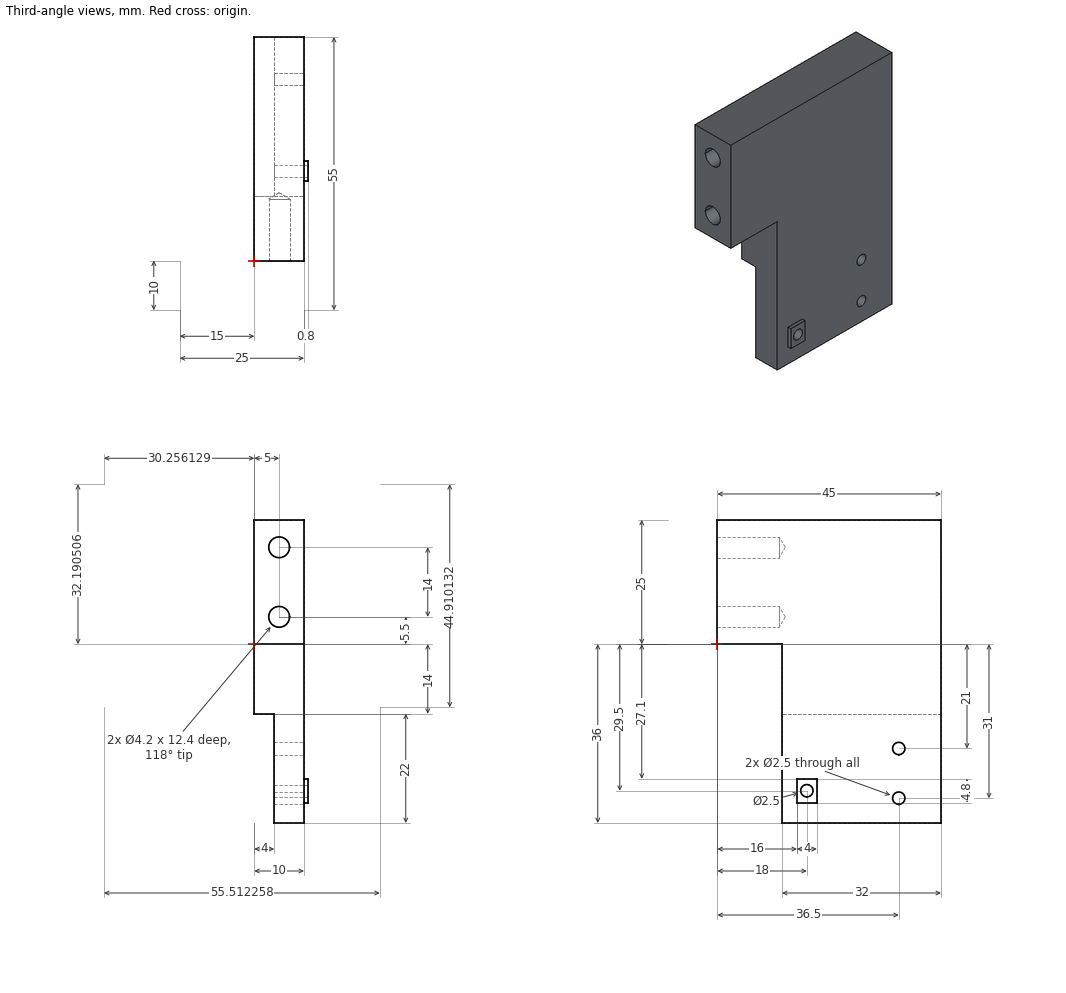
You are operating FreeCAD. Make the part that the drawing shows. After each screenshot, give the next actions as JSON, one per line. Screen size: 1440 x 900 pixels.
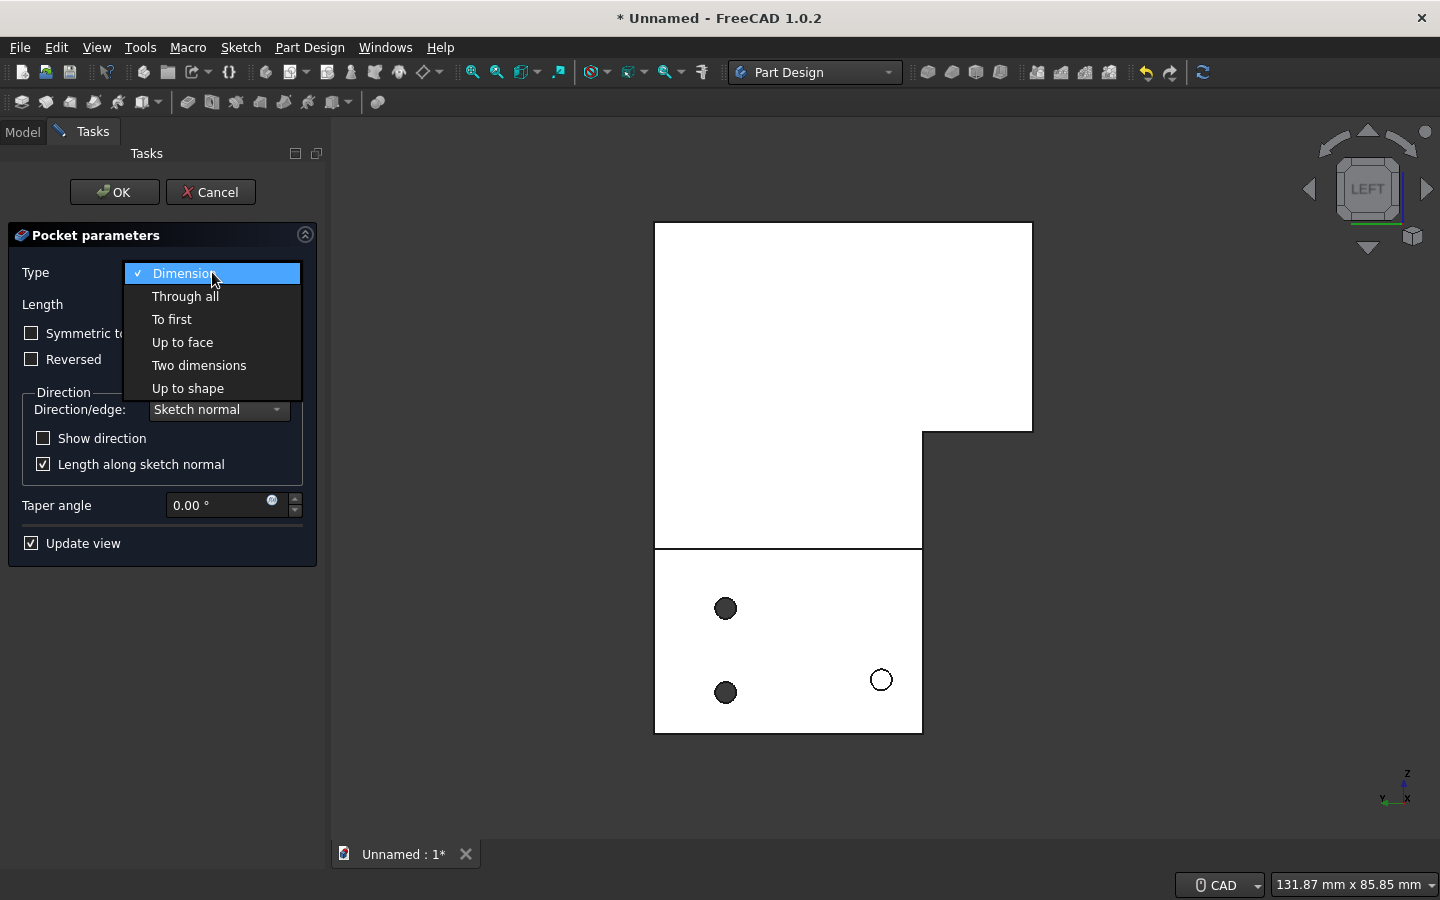
{"action": "left_click", "coordinate": [212, 296]}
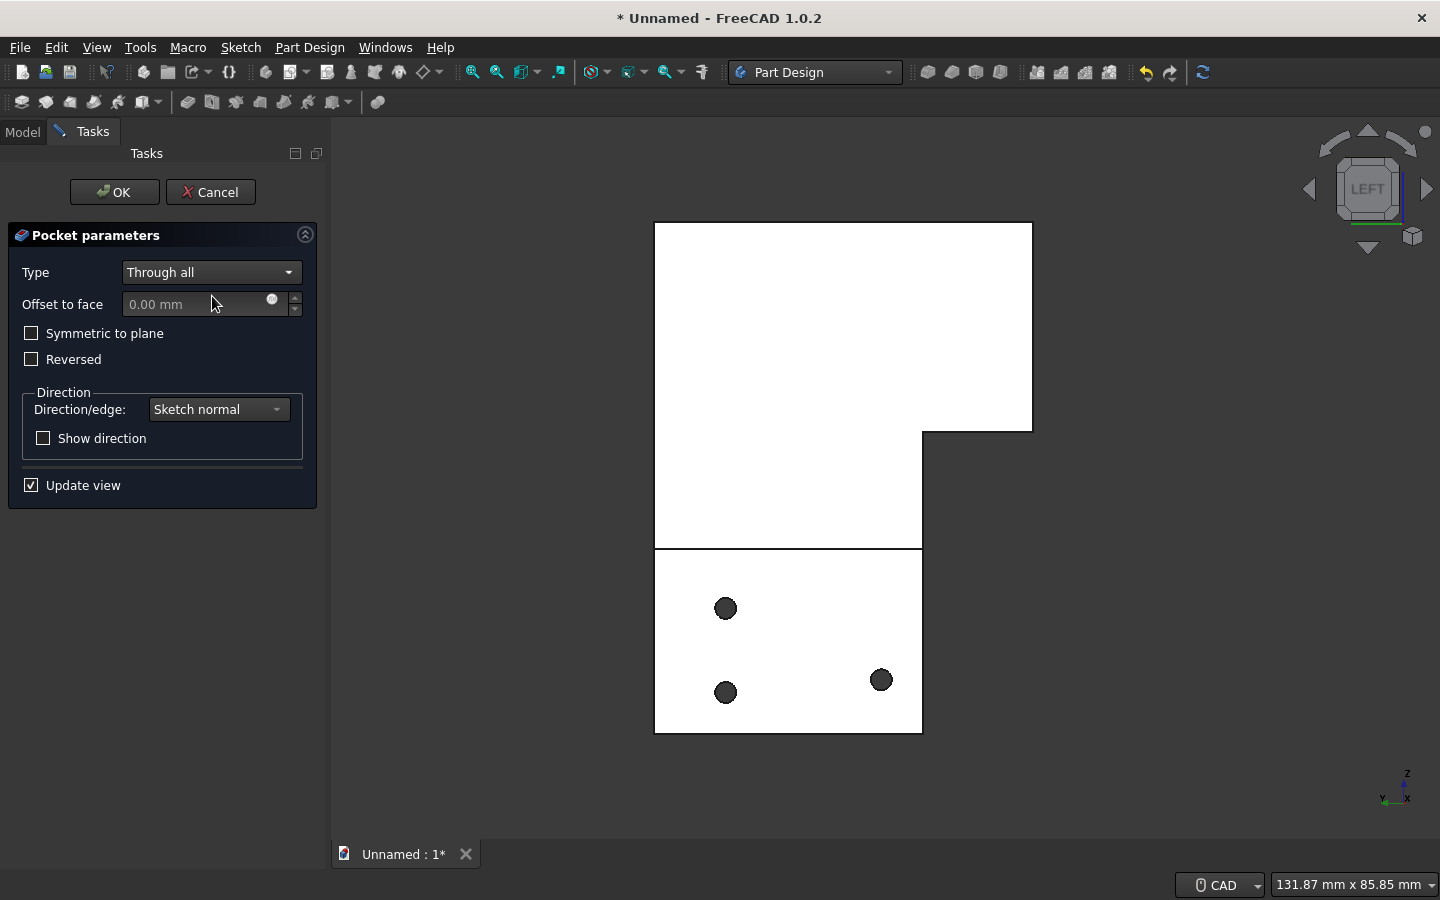
{"action": "left_click", "coordinate": [115, 192]}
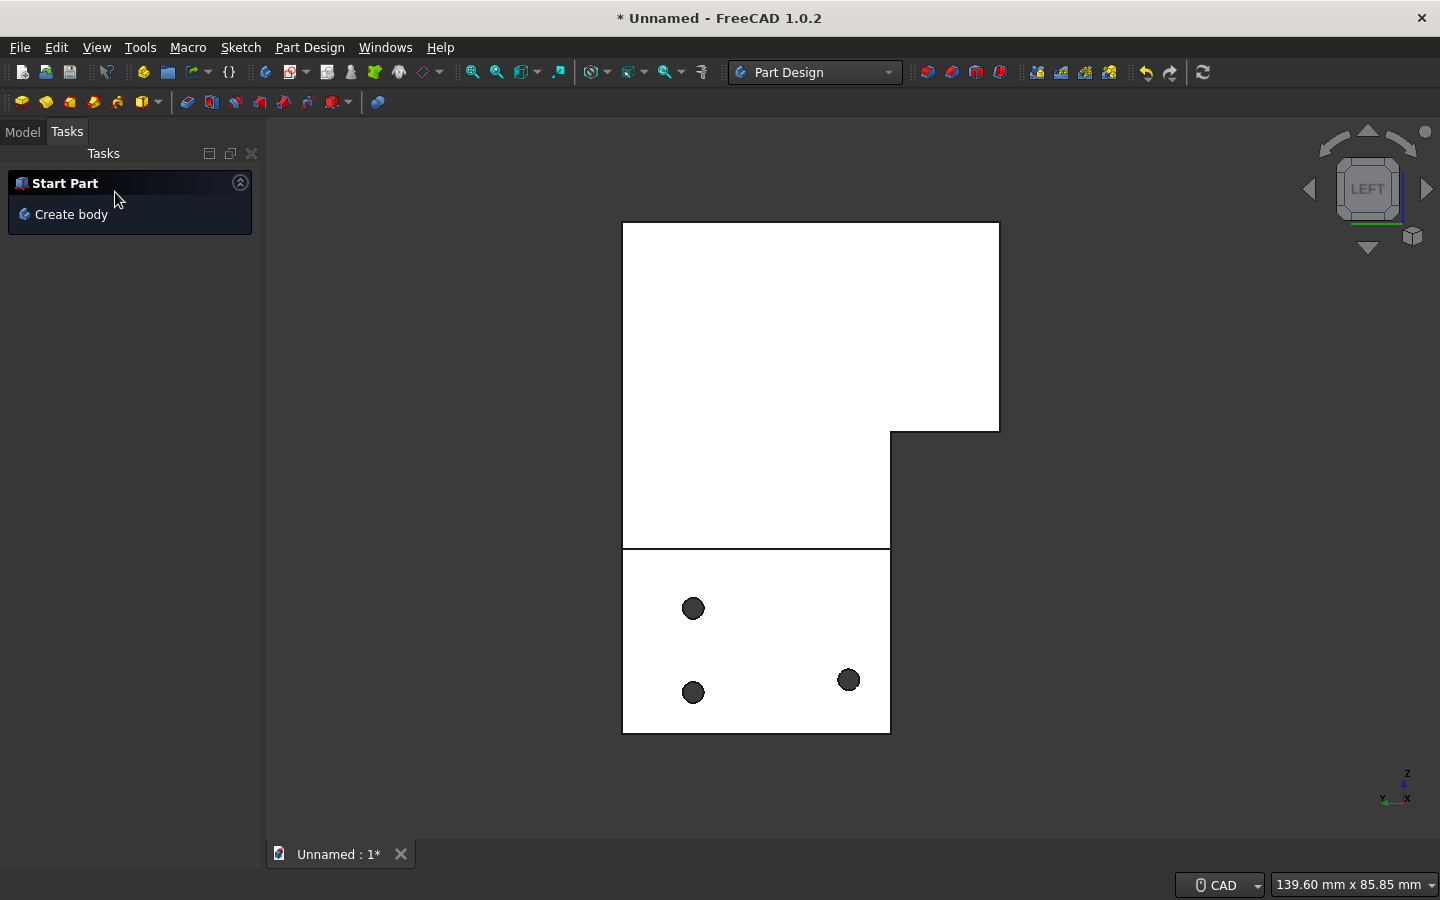
{"action": "key", "text": "0"}